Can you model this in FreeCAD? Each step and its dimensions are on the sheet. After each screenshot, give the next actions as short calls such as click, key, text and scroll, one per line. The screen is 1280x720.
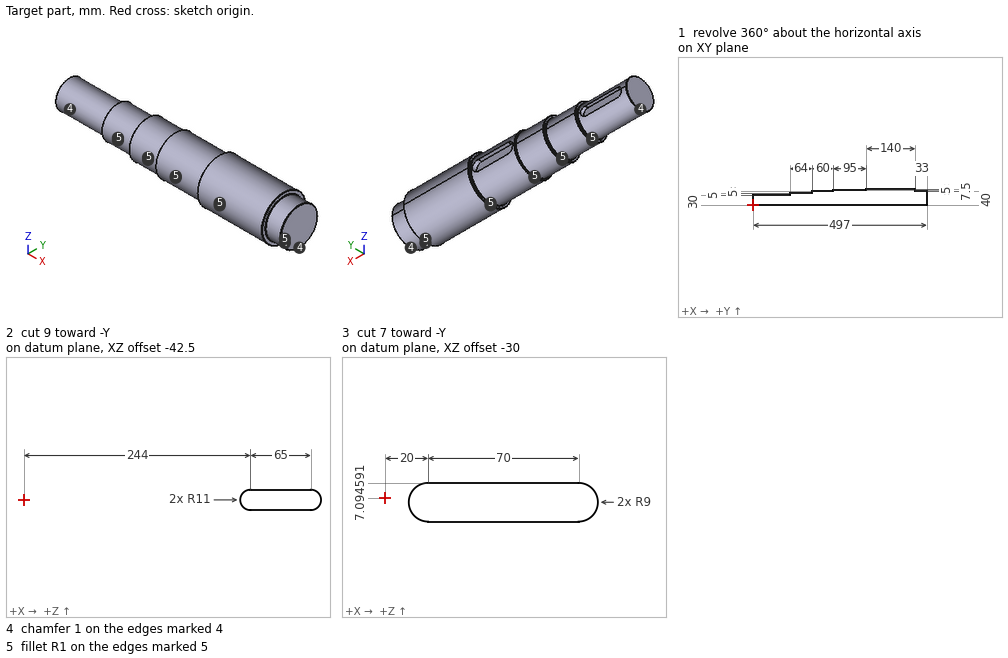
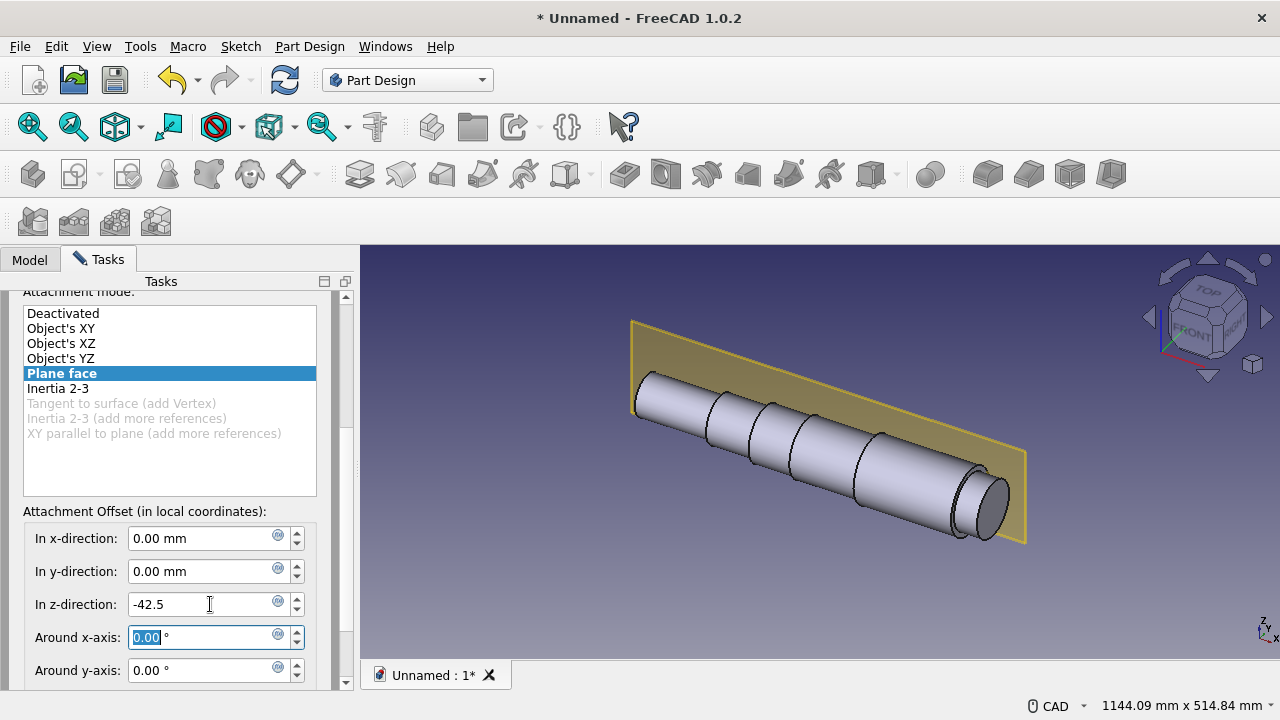
scroll(346, 490, up, 5)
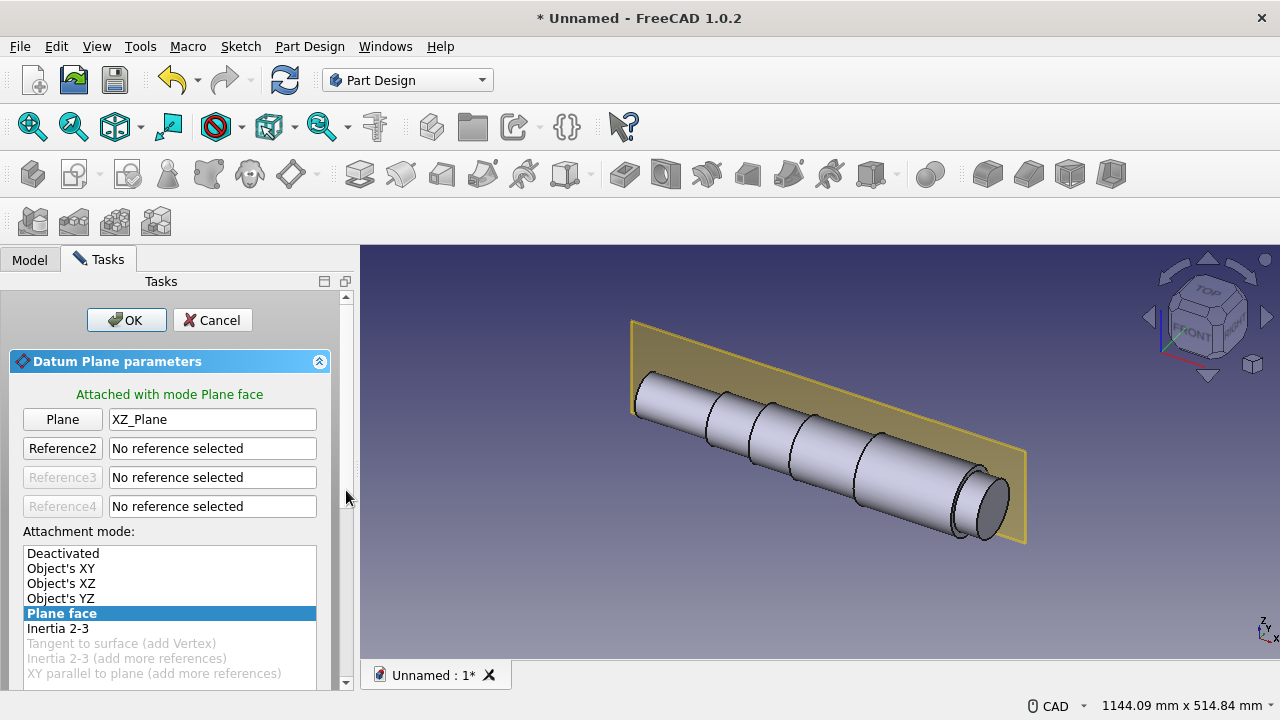
click(127, 320)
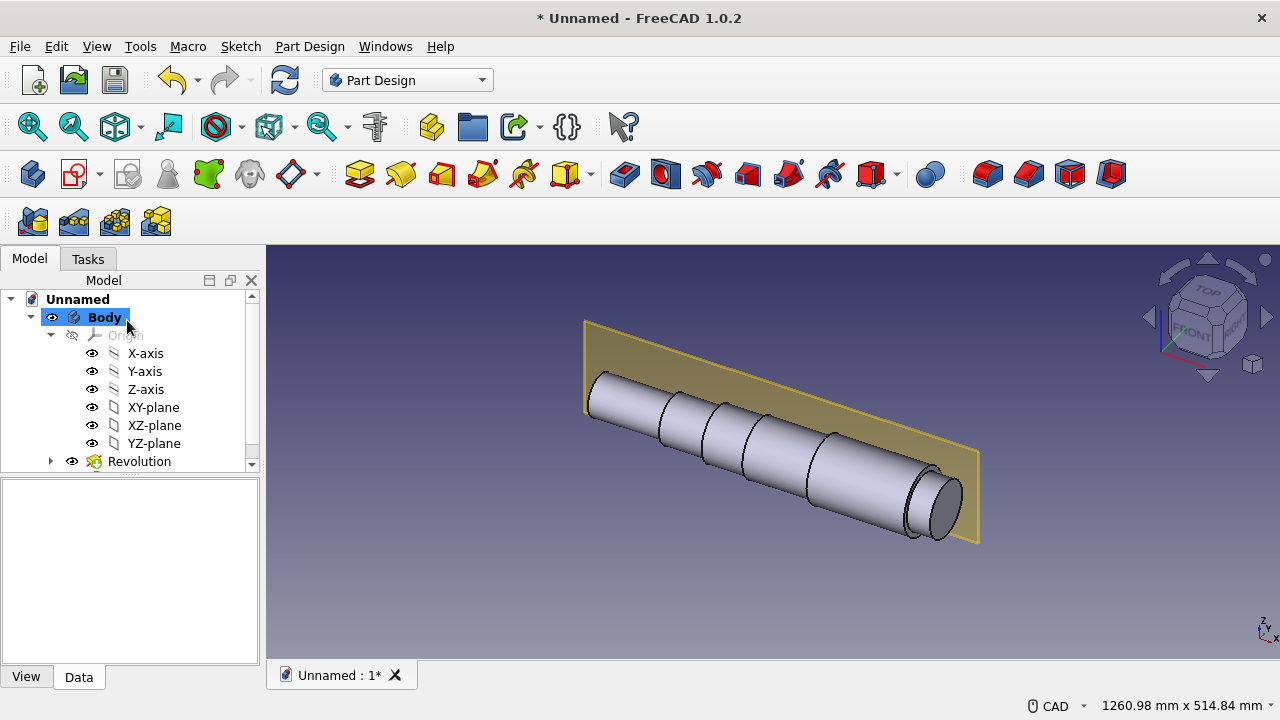
scroll(101, 385, down, 3)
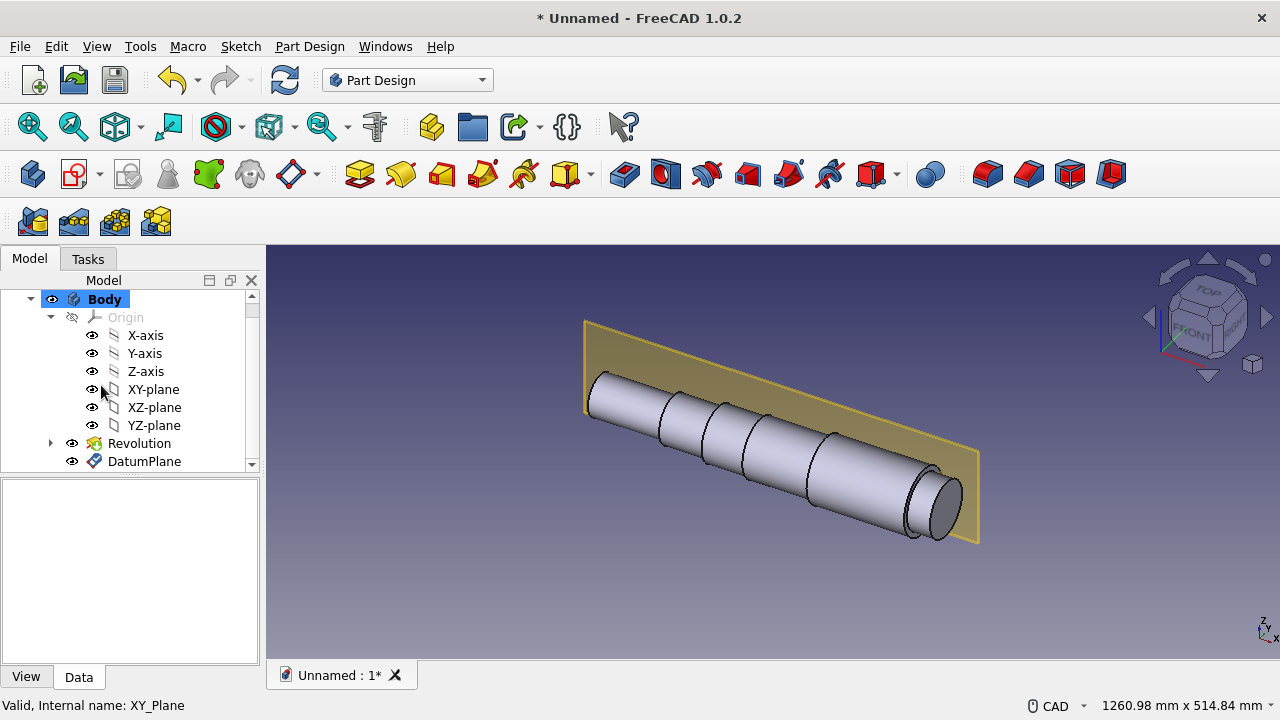
click(117, 461)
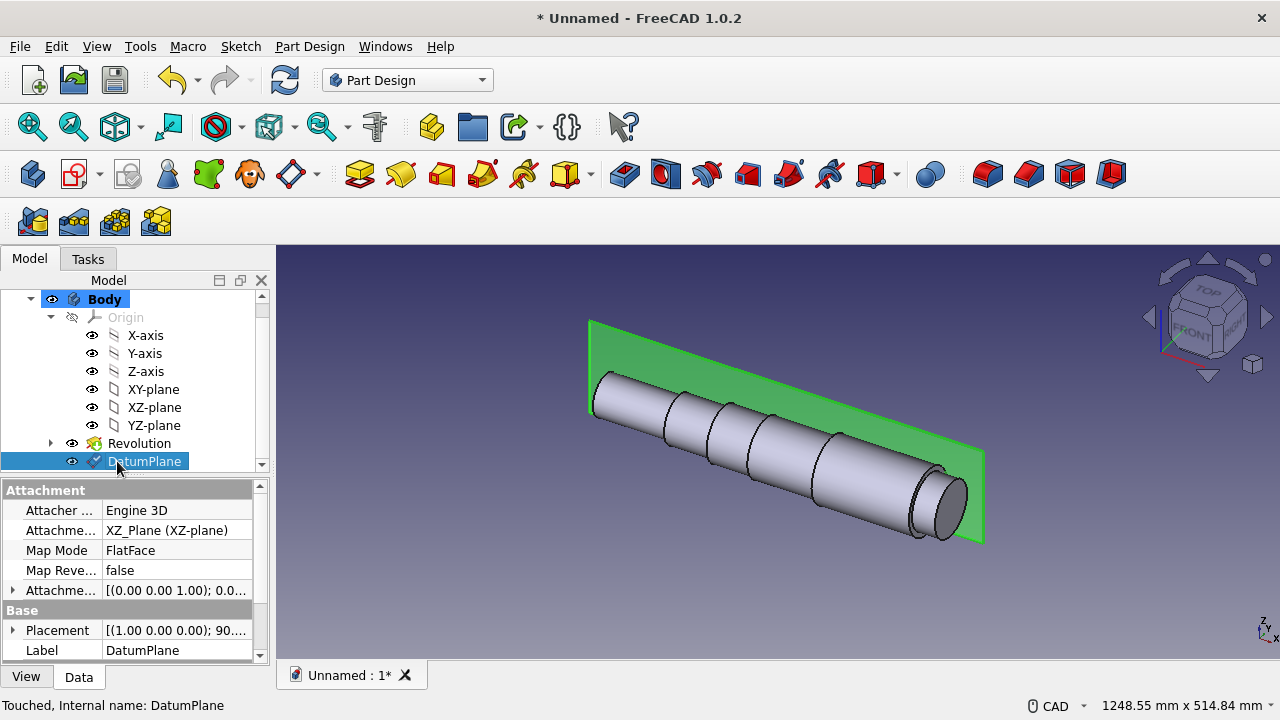
click(74, 174)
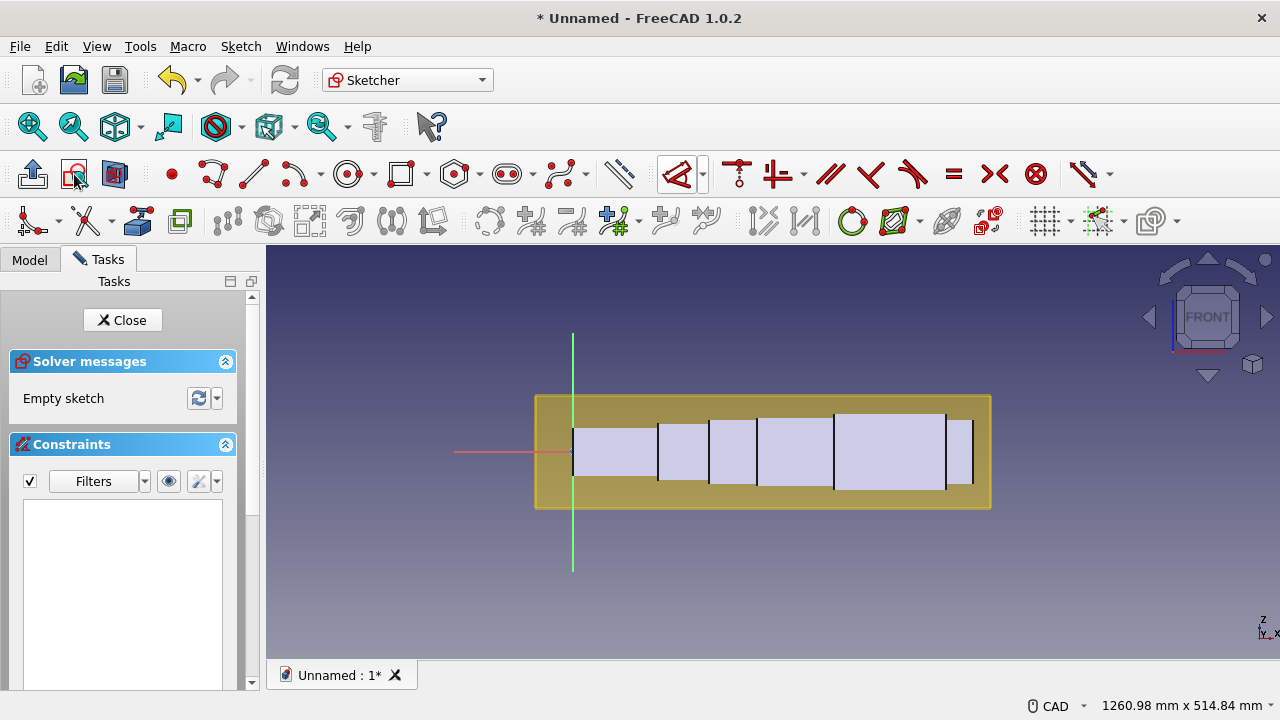
click(115, 174)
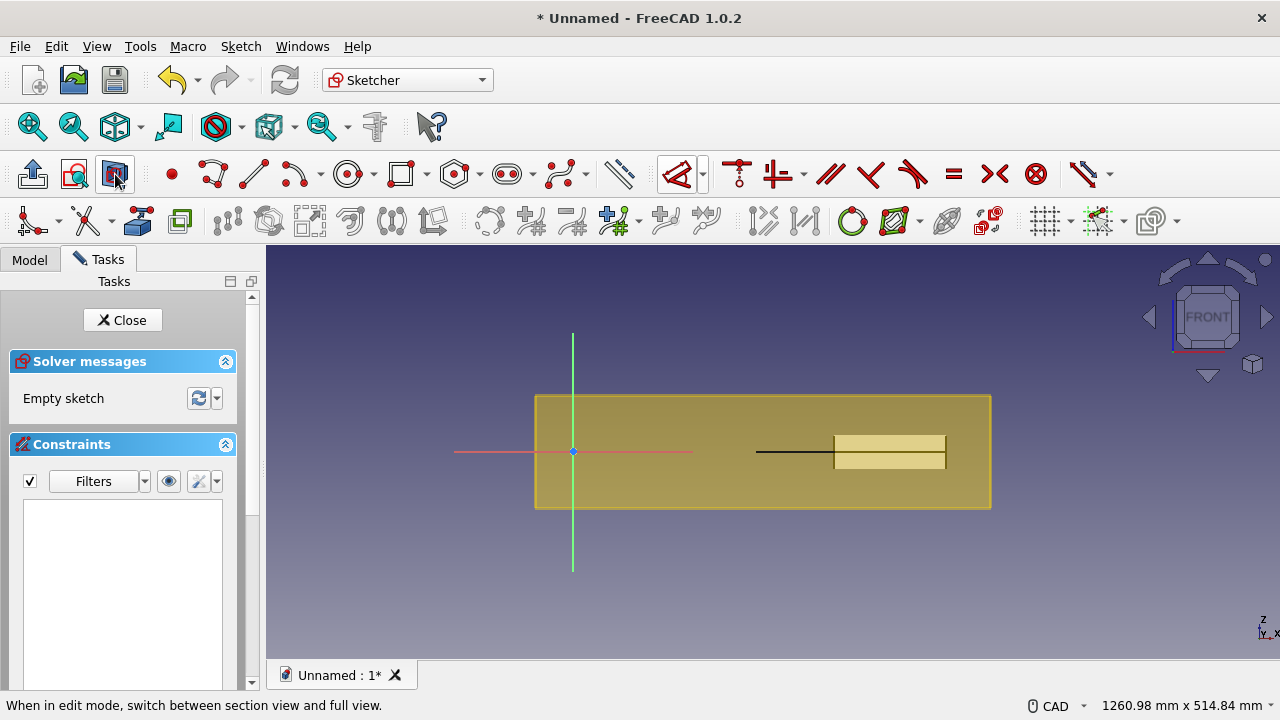
scroll(807, 452, up, 11)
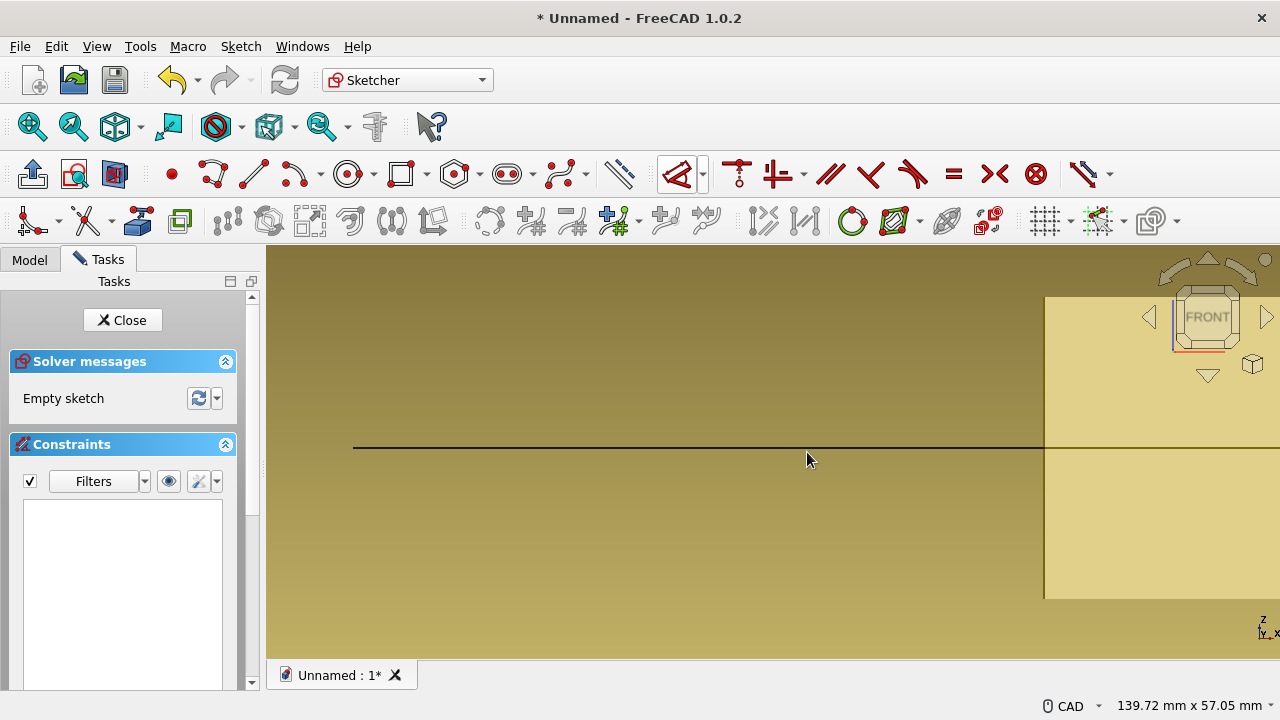
click(506, 174)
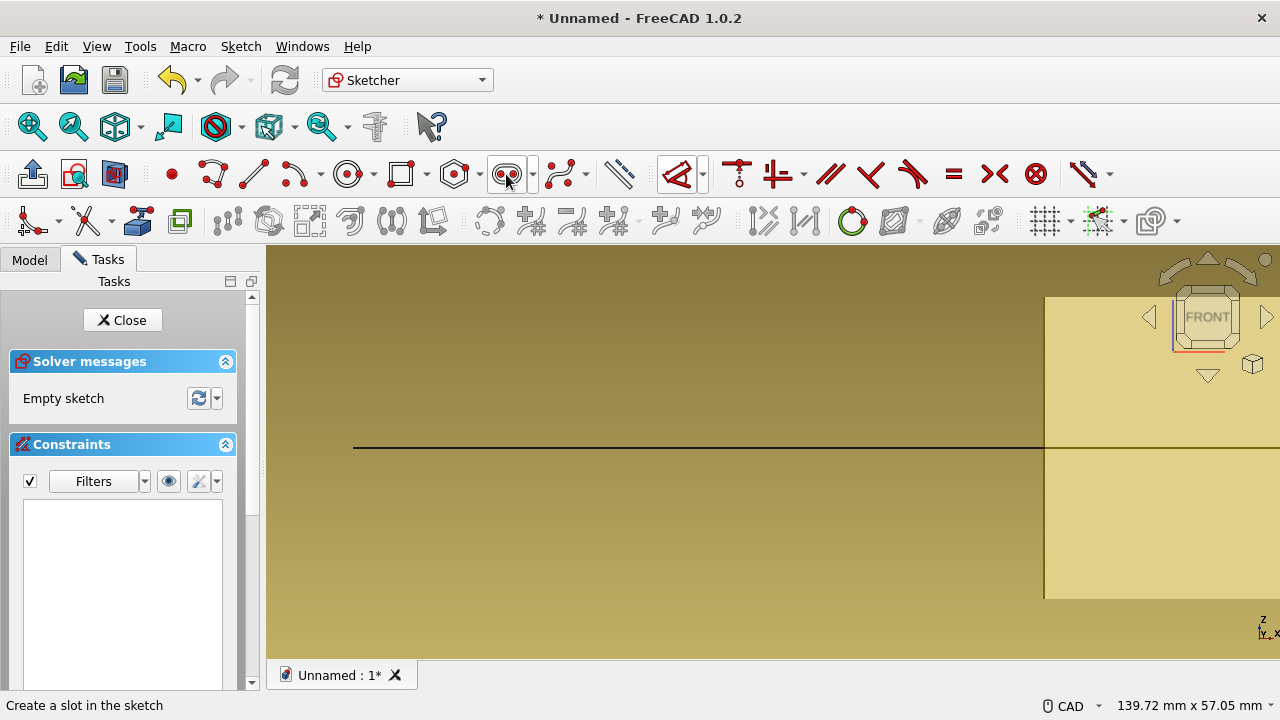
click(463, 448)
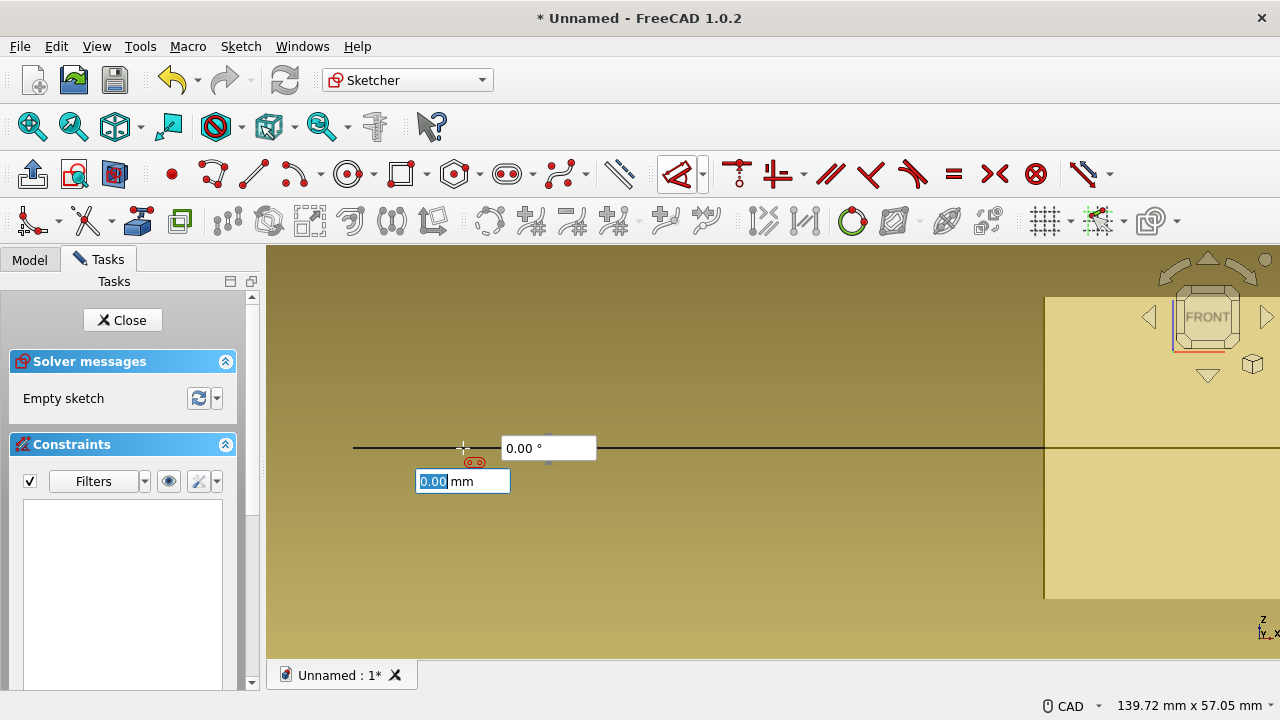
click(935, 439)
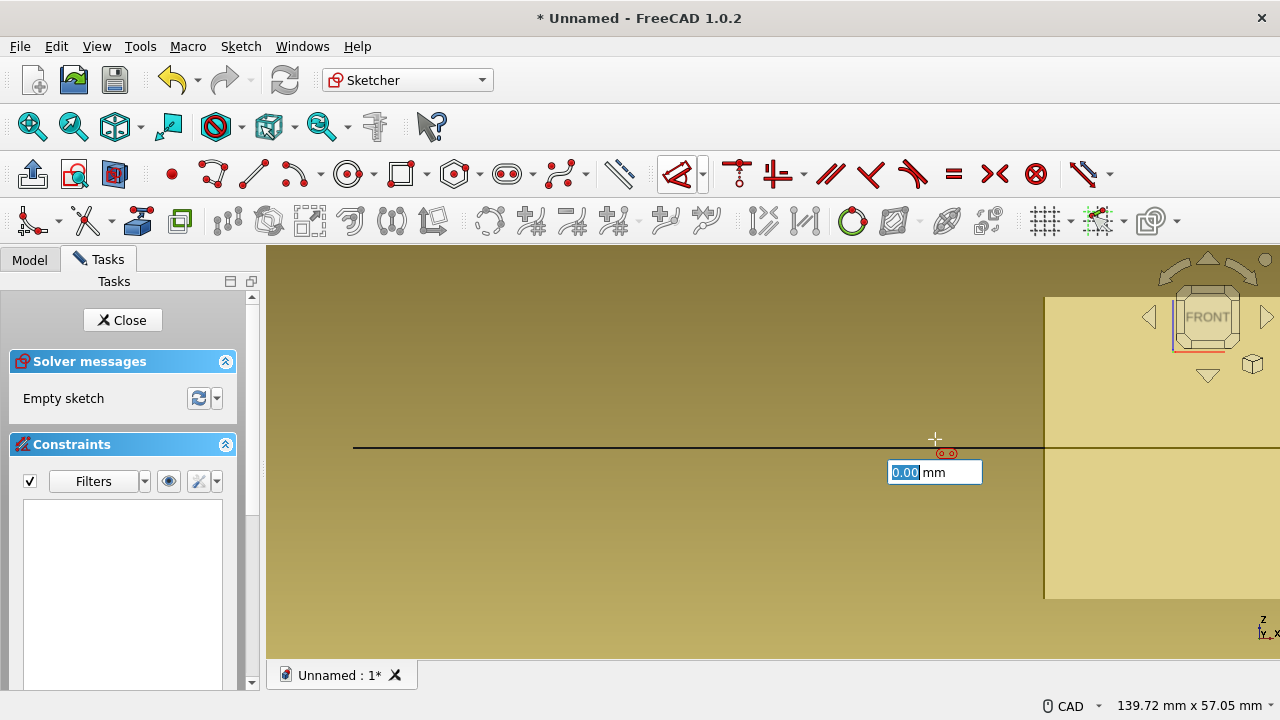
click(699, 528)
key(Escape)